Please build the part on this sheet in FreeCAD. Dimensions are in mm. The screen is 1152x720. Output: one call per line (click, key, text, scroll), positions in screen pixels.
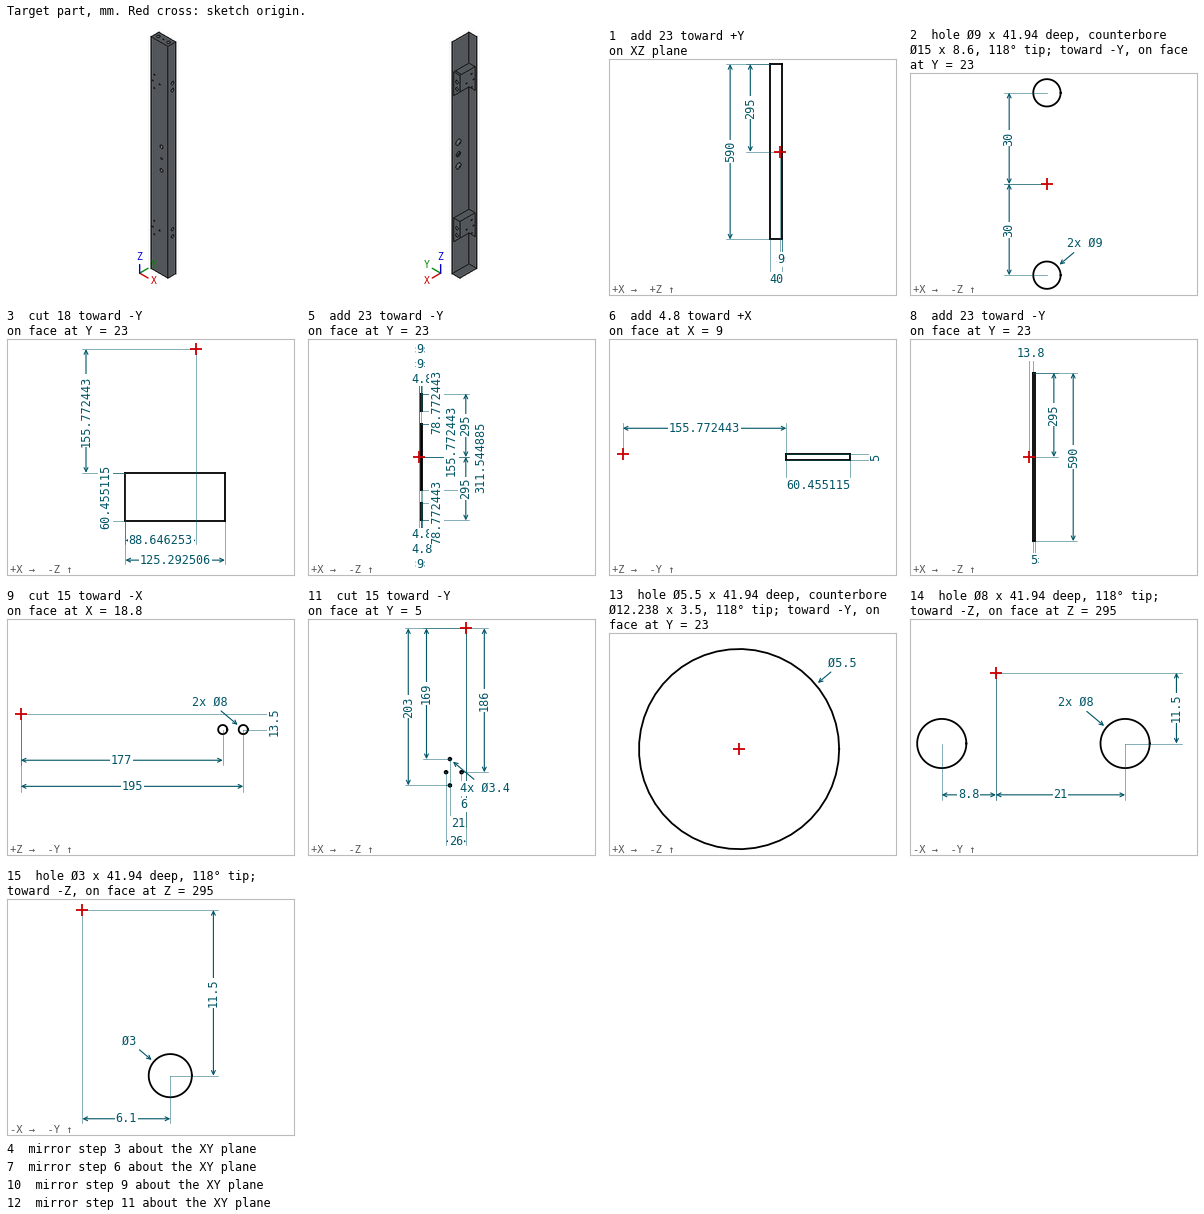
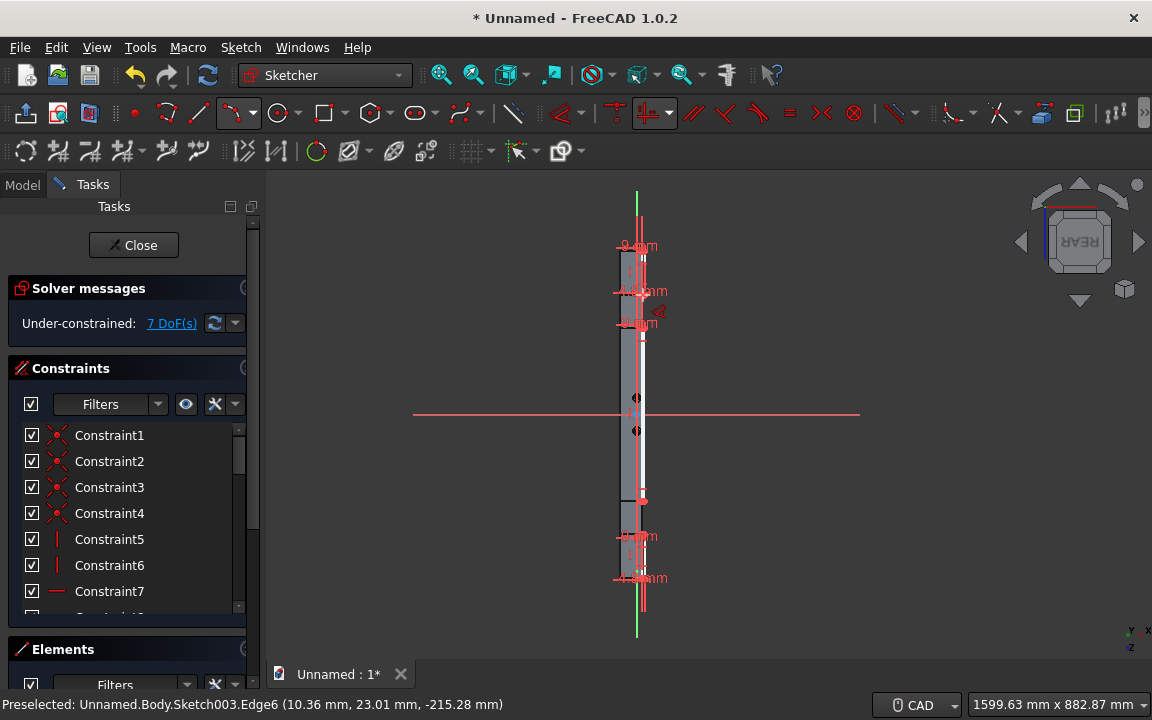
scroll(643, 501, up, 14)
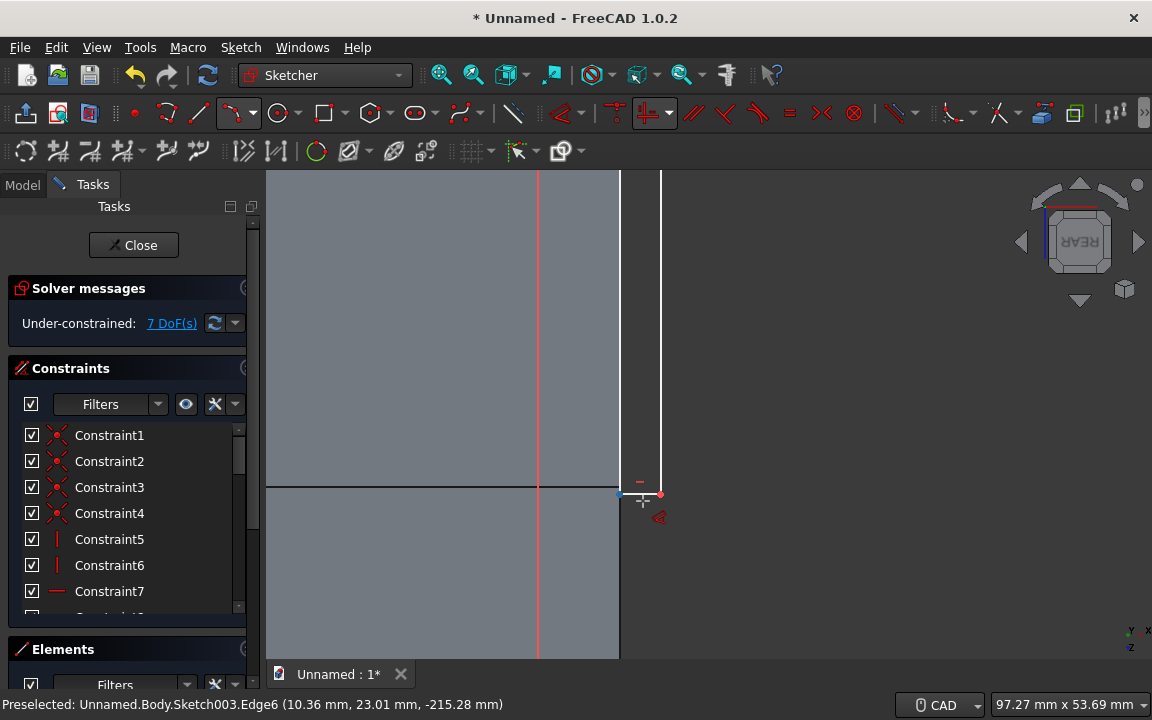
click(632, 494)
click(640, 528)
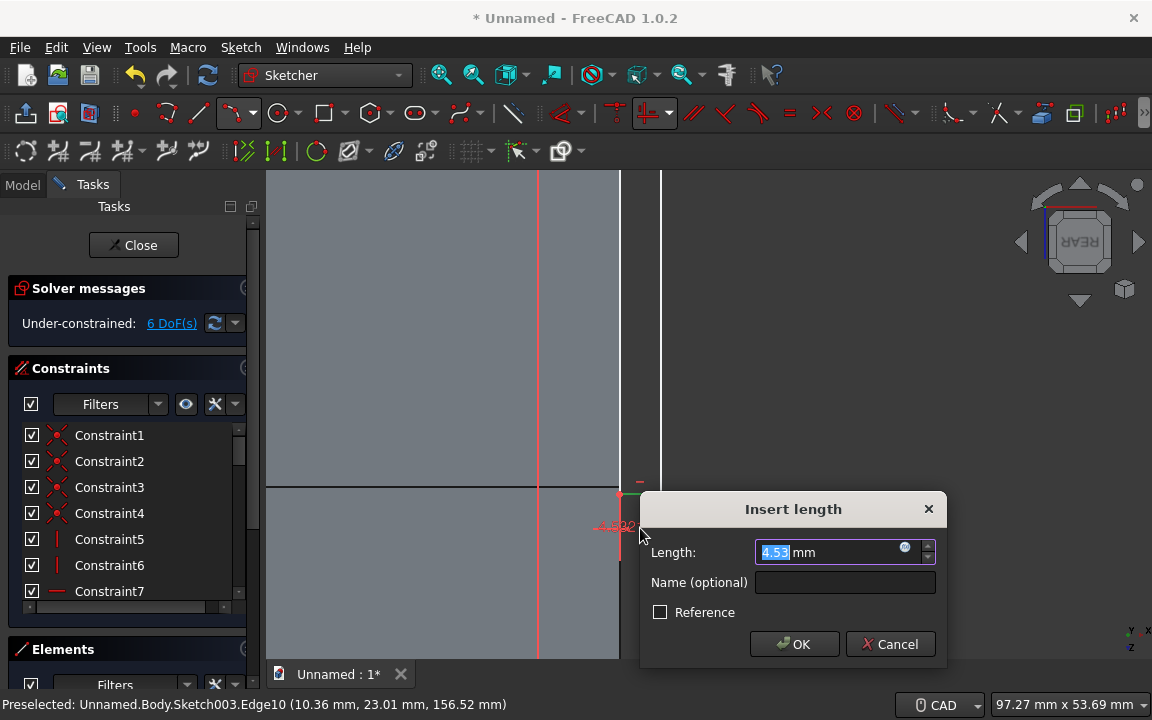
text(4.8)
key(Return)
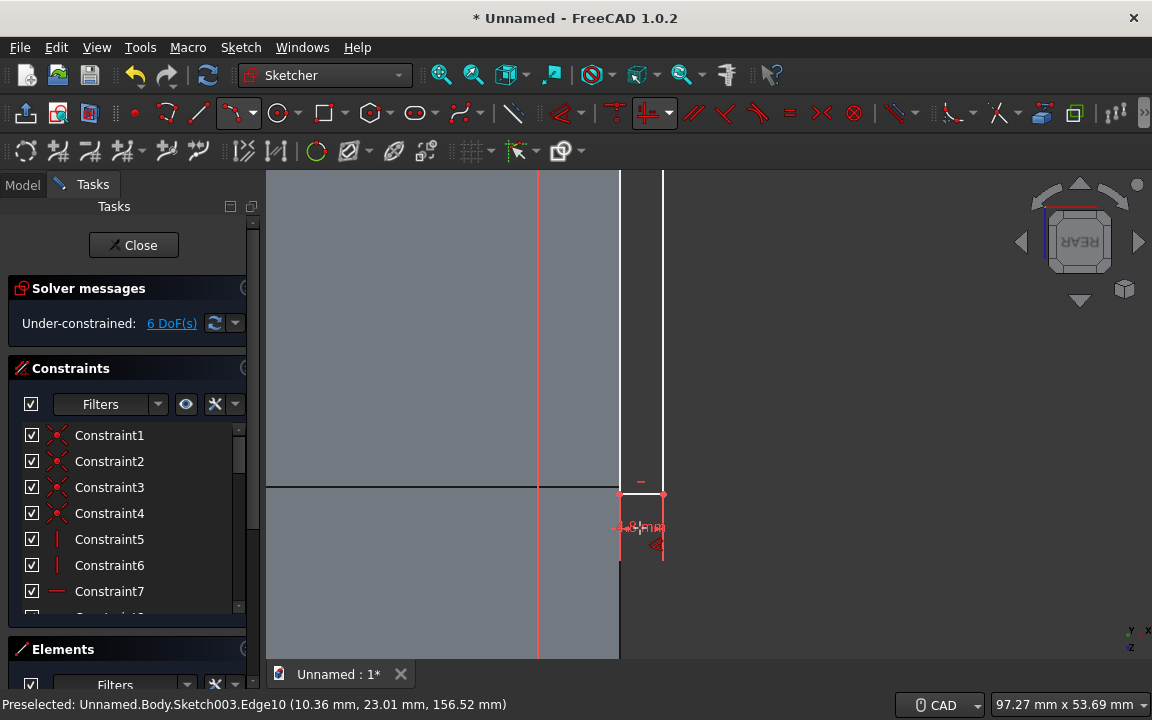
scroll(643, 502, down, 14)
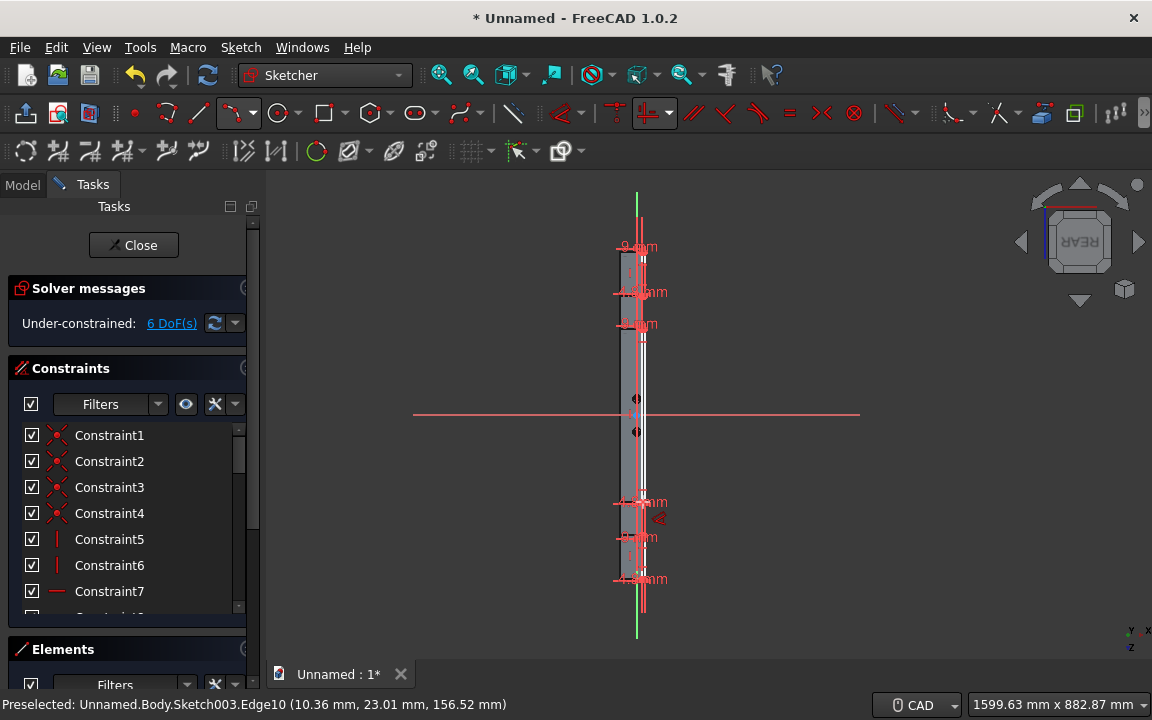
scroll(642, 579, up, 8)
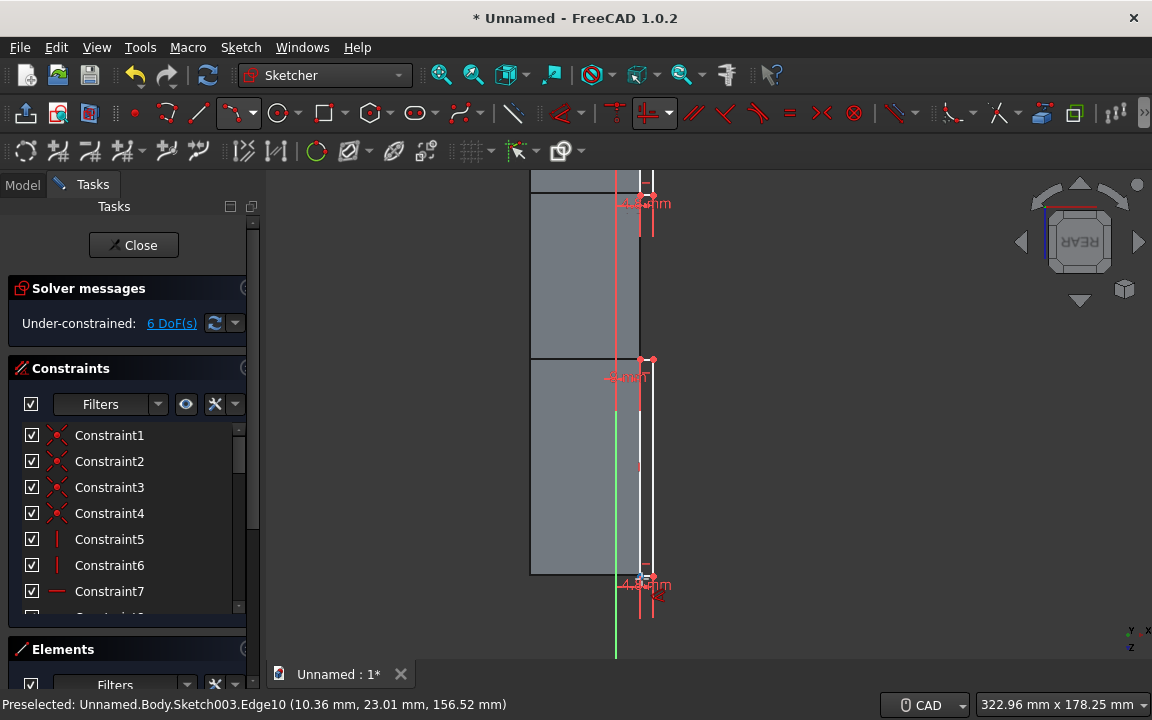
click(640, 576)
click(582, 300)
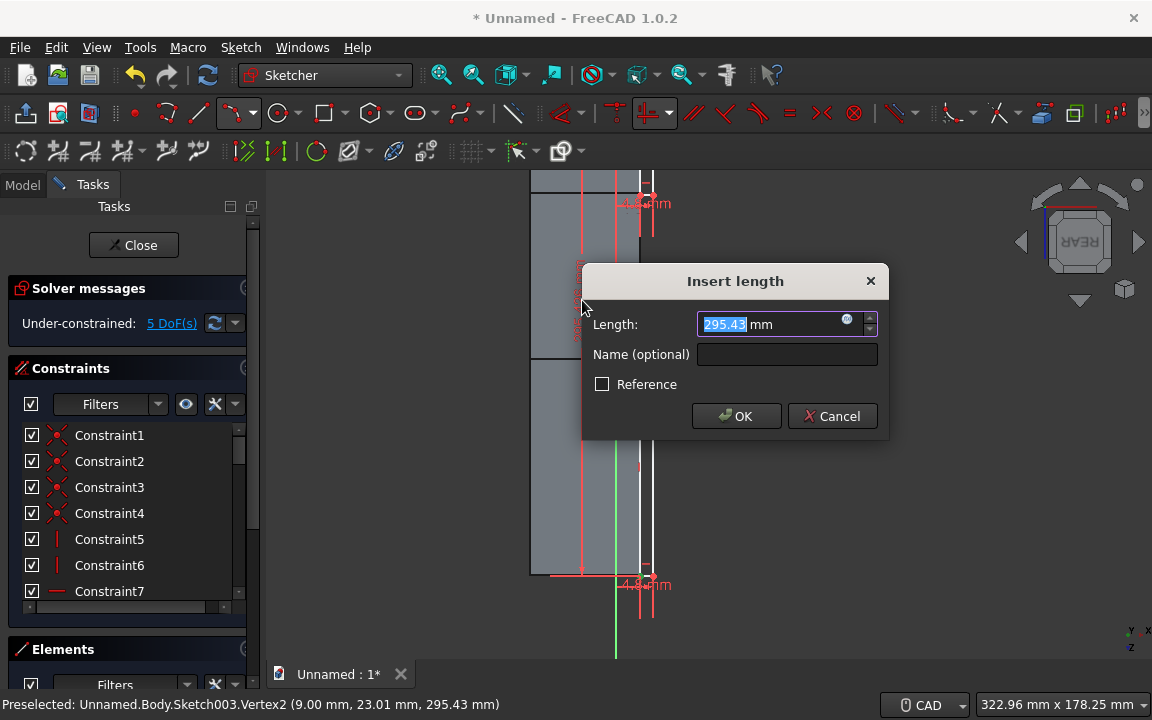
text(295)
key(Return)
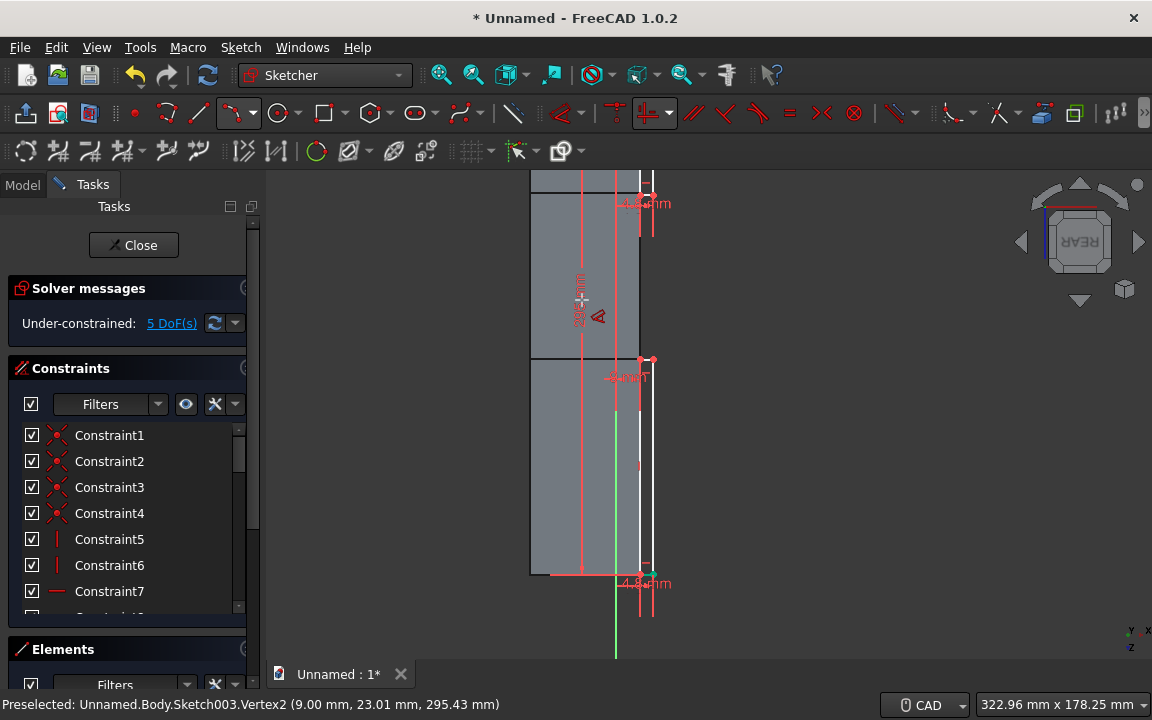
scroll(642, 579, down, 8)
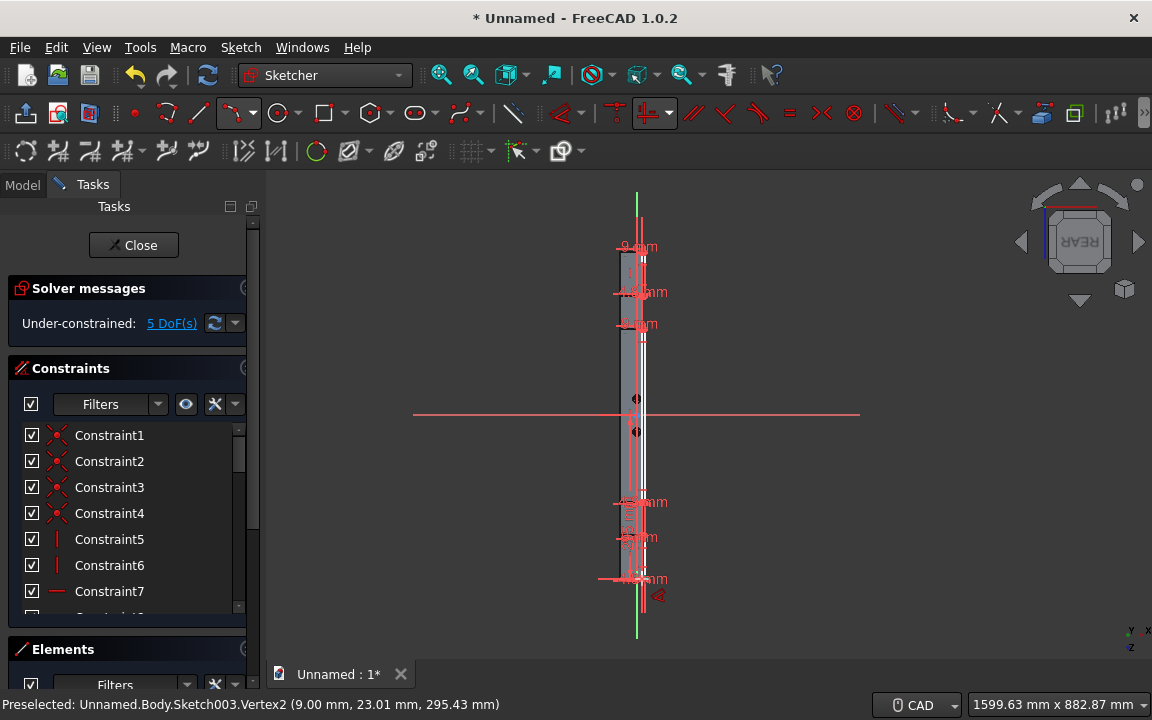
scroll(642, 252, up, 8)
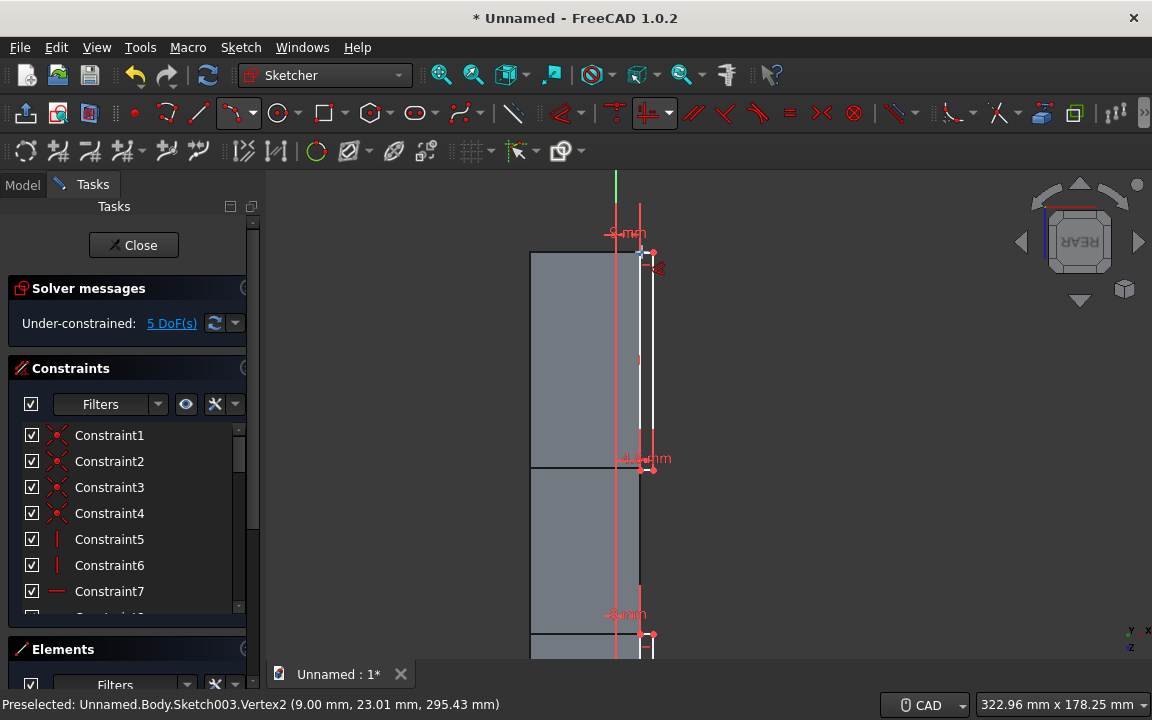
click(640, 253)
click(582, 355)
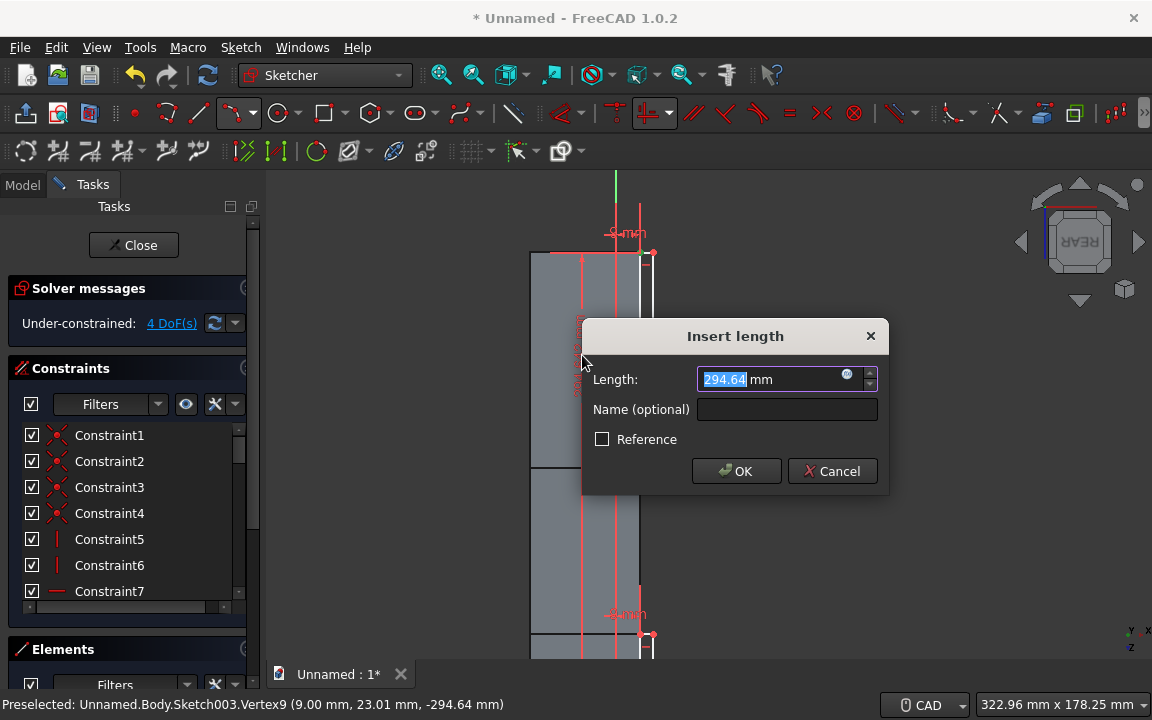
text(295)
key(Return)